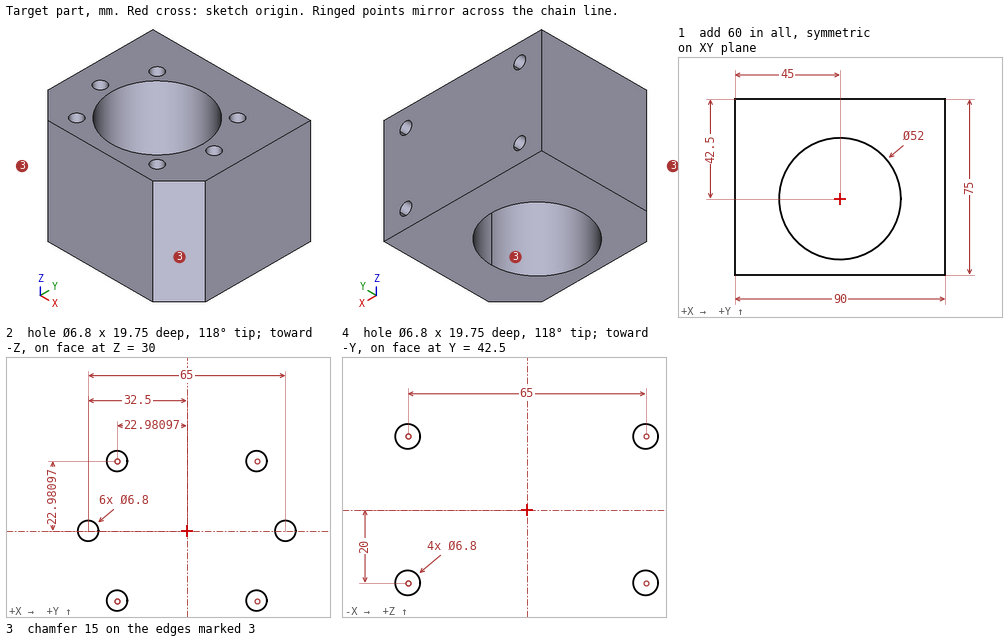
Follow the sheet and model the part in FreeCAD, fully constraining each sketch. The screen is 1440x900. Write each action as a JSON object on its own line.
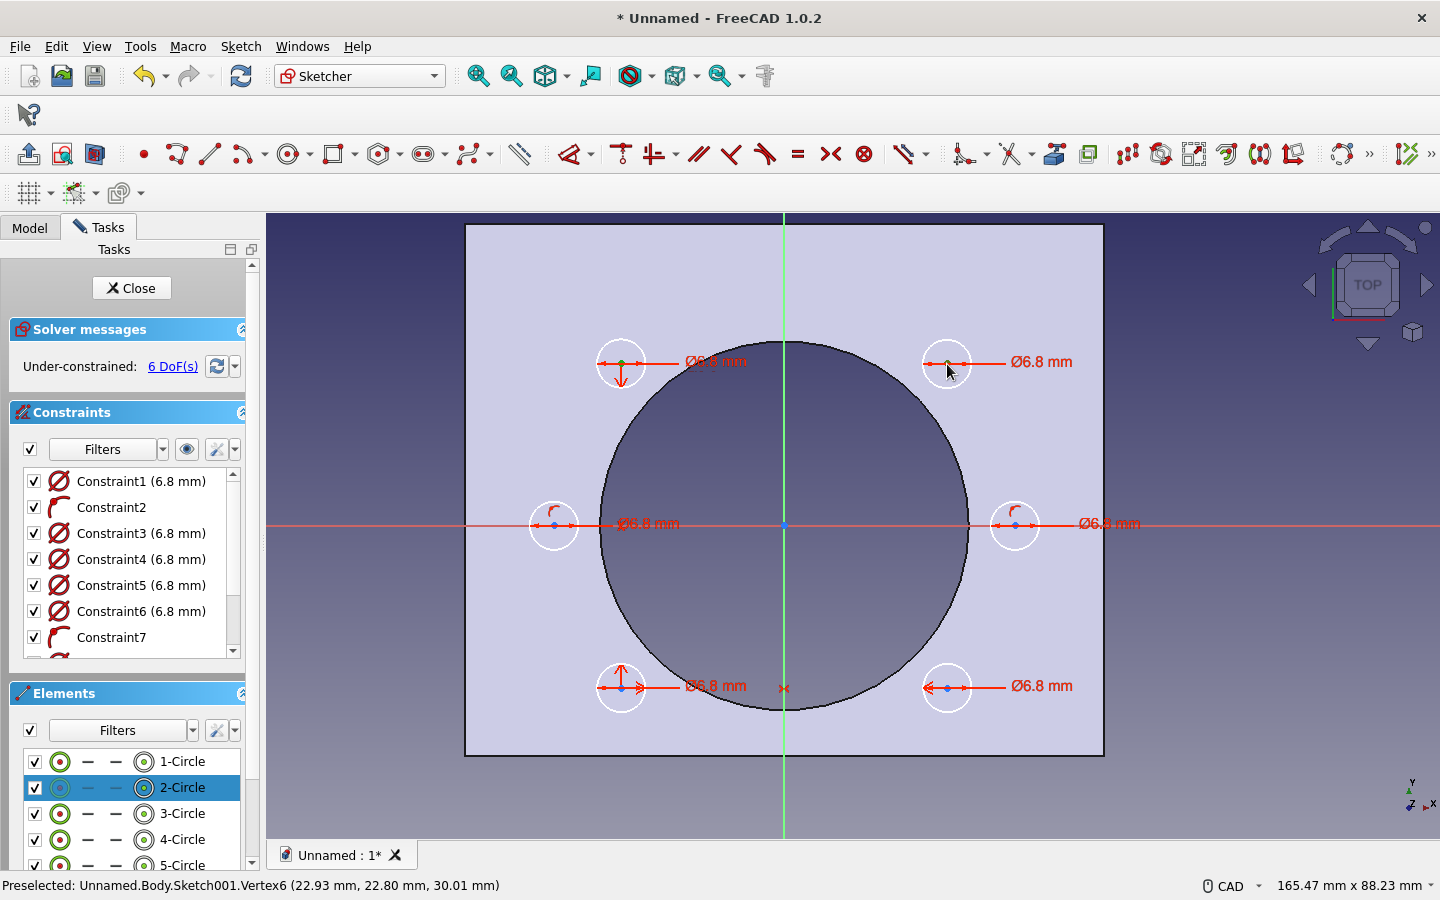
{"action": "left_click", "coordinate": [784, 770]}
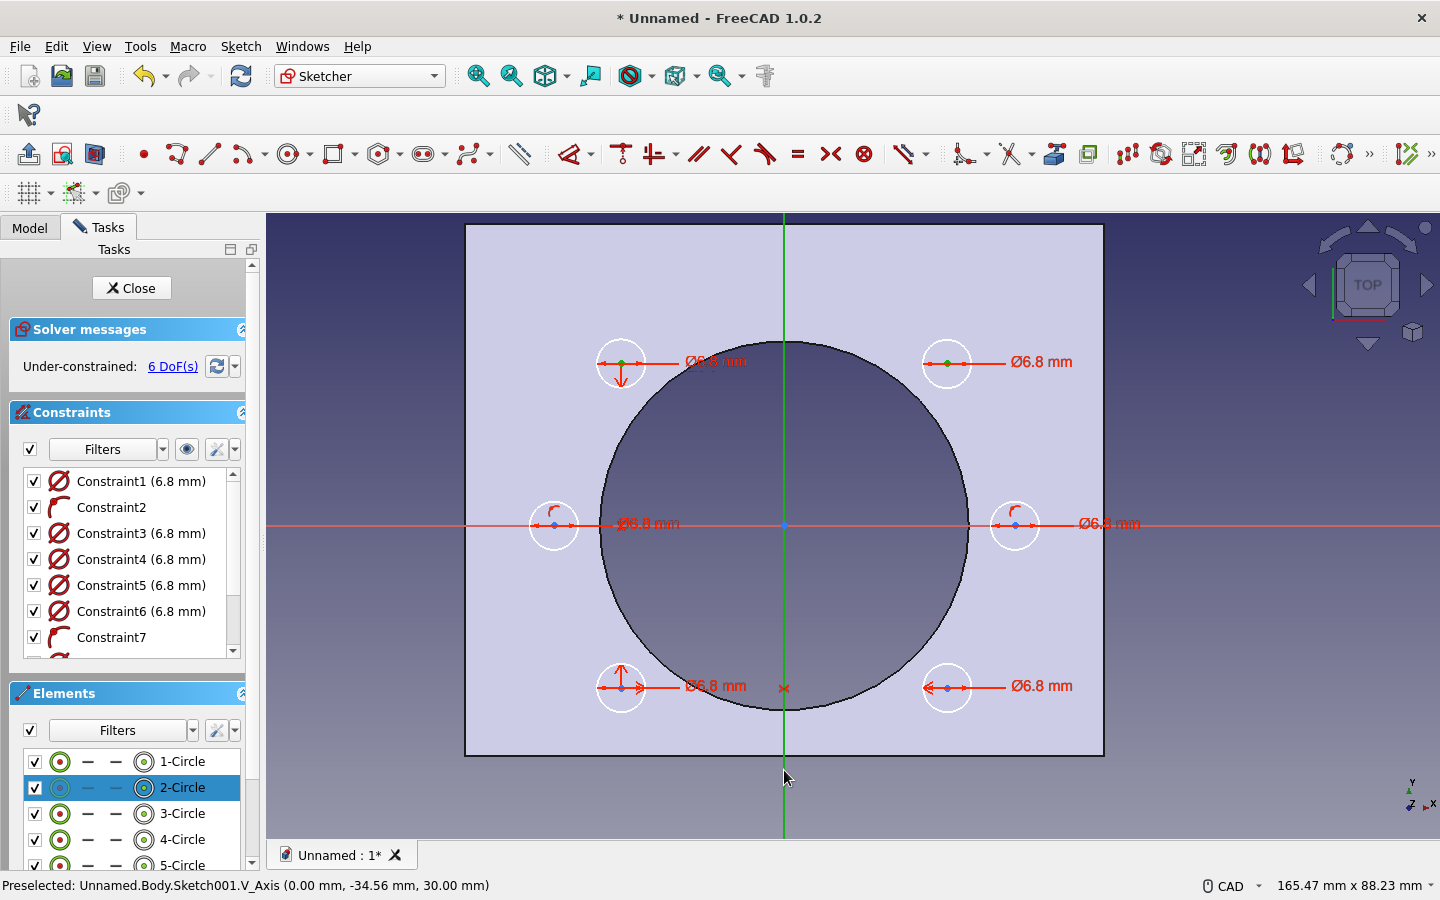
{"action": "left_click", "coordinate": [831, 154]}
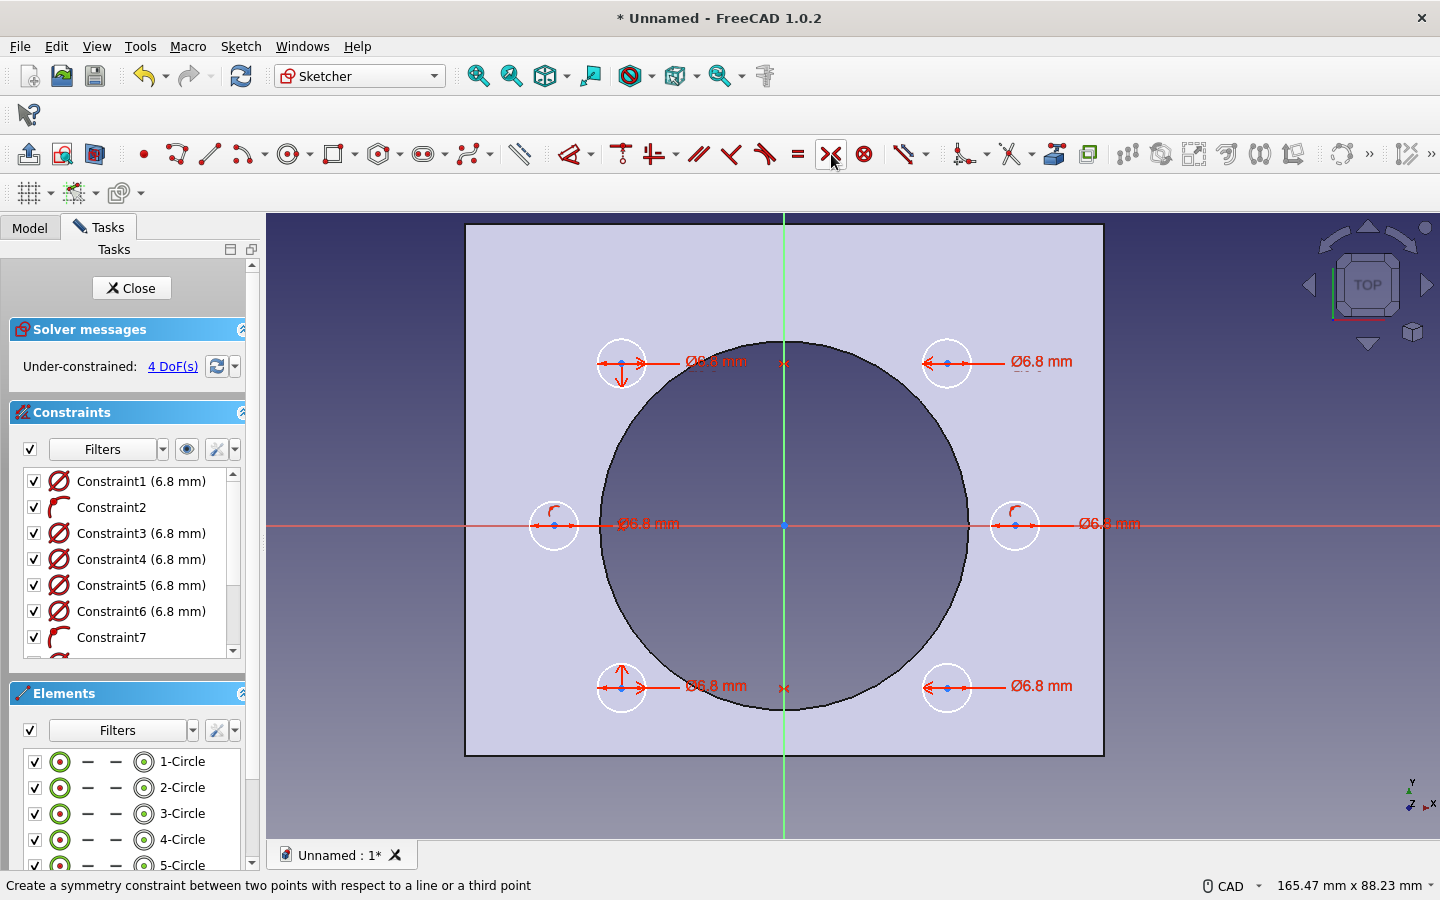
{"action": "left_click", "coordinate": [568, 154]}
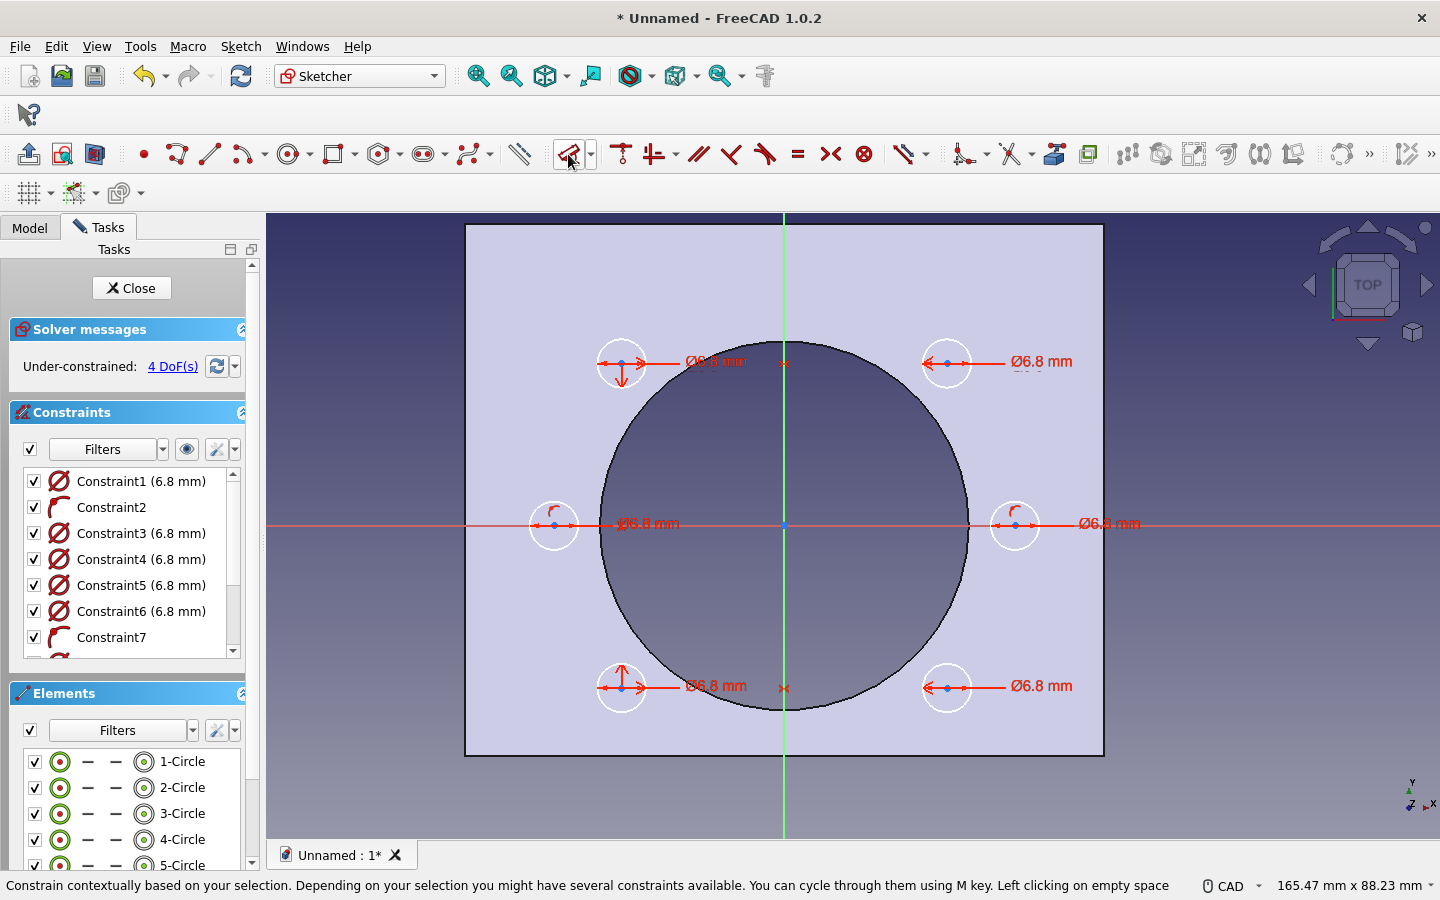
{"action": "left_click", "coordinate": [554, 526]}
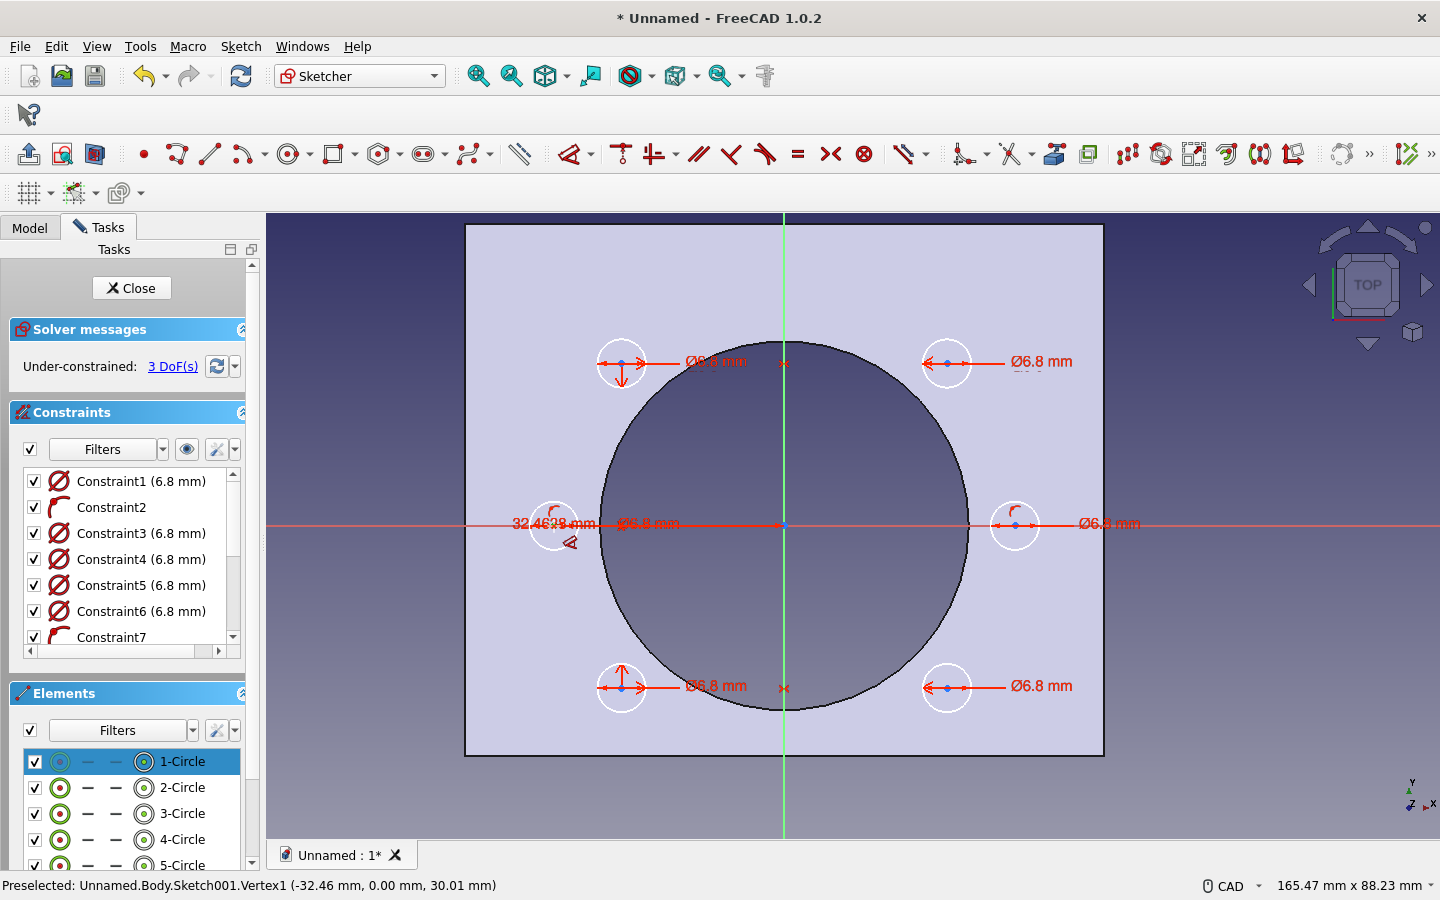
{"action": "left_click", "coordinate": [1015, 526]}
{"action": "left_click", "coordinate": [678, 560]}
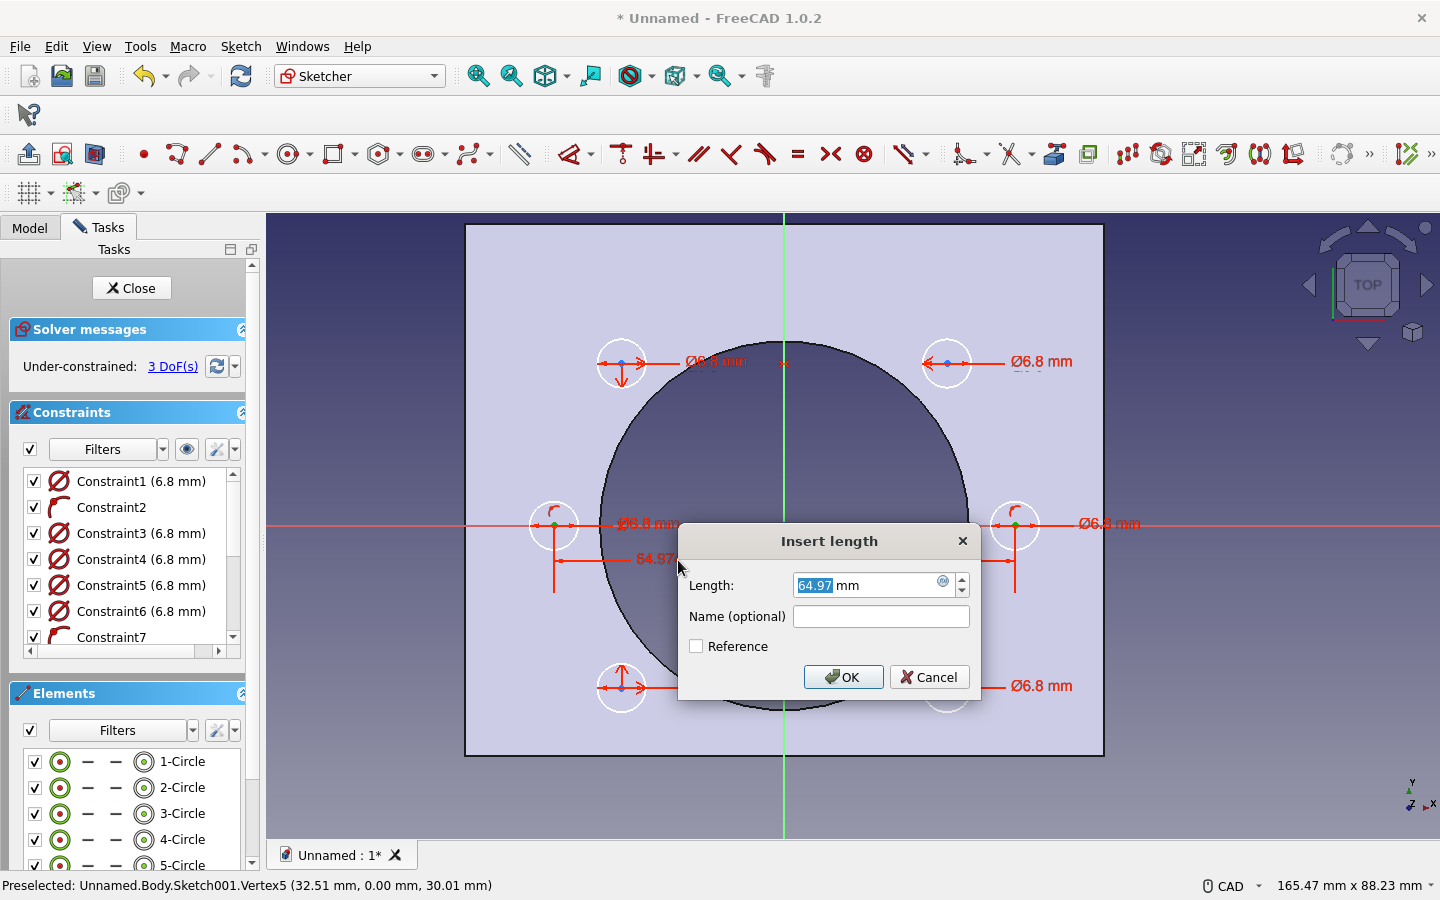
{"action": "type", "text": "65"}
{"action": "key", "text": "Return"}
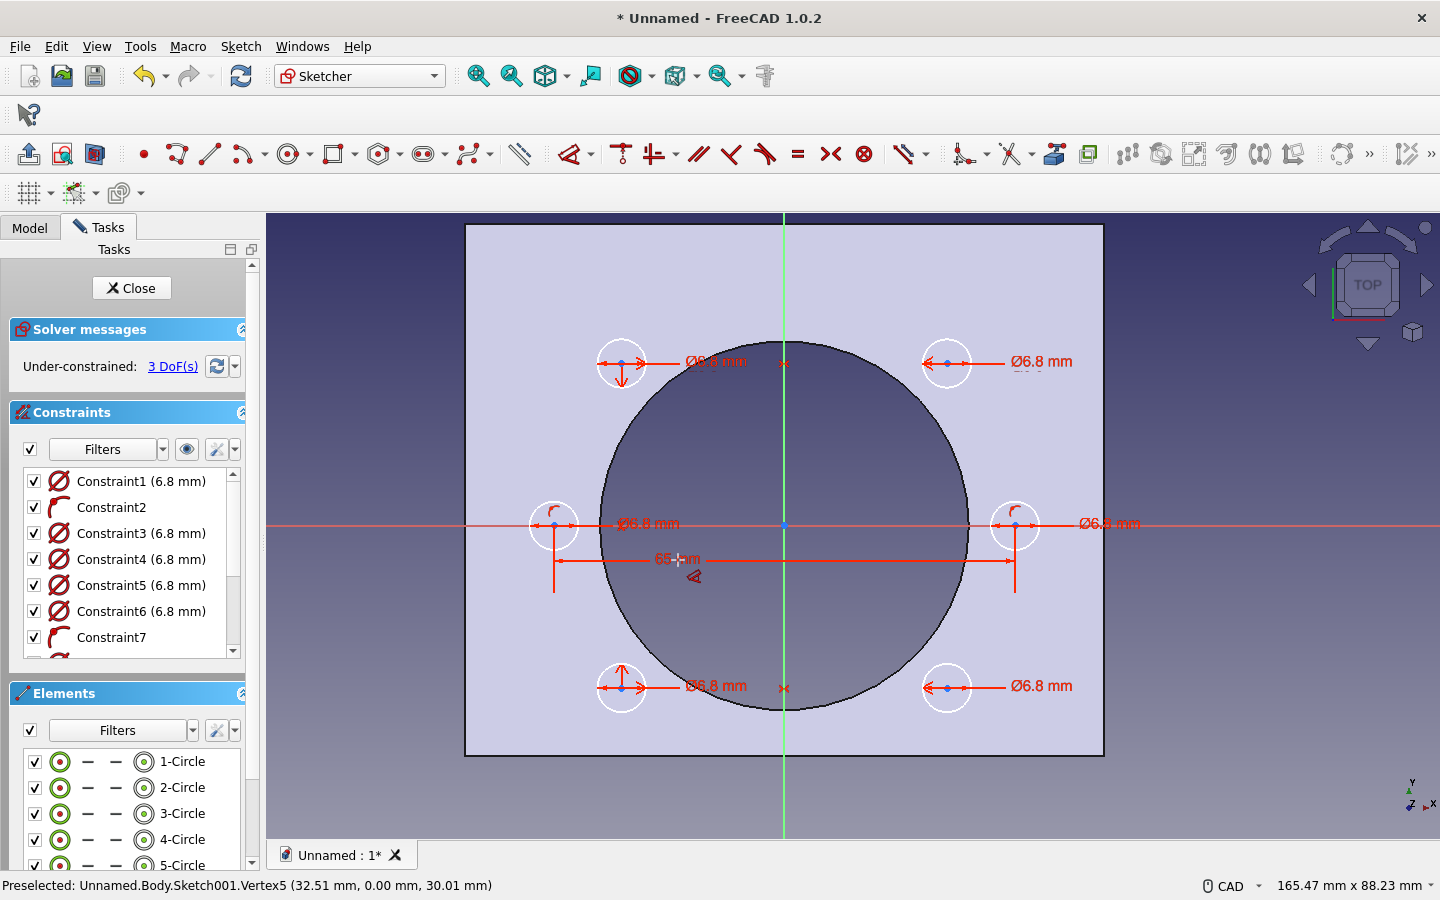
{"action": "left_click", "coordinate": [554, 526]}
{"action": "left_click", "coordinate": [589, 560]}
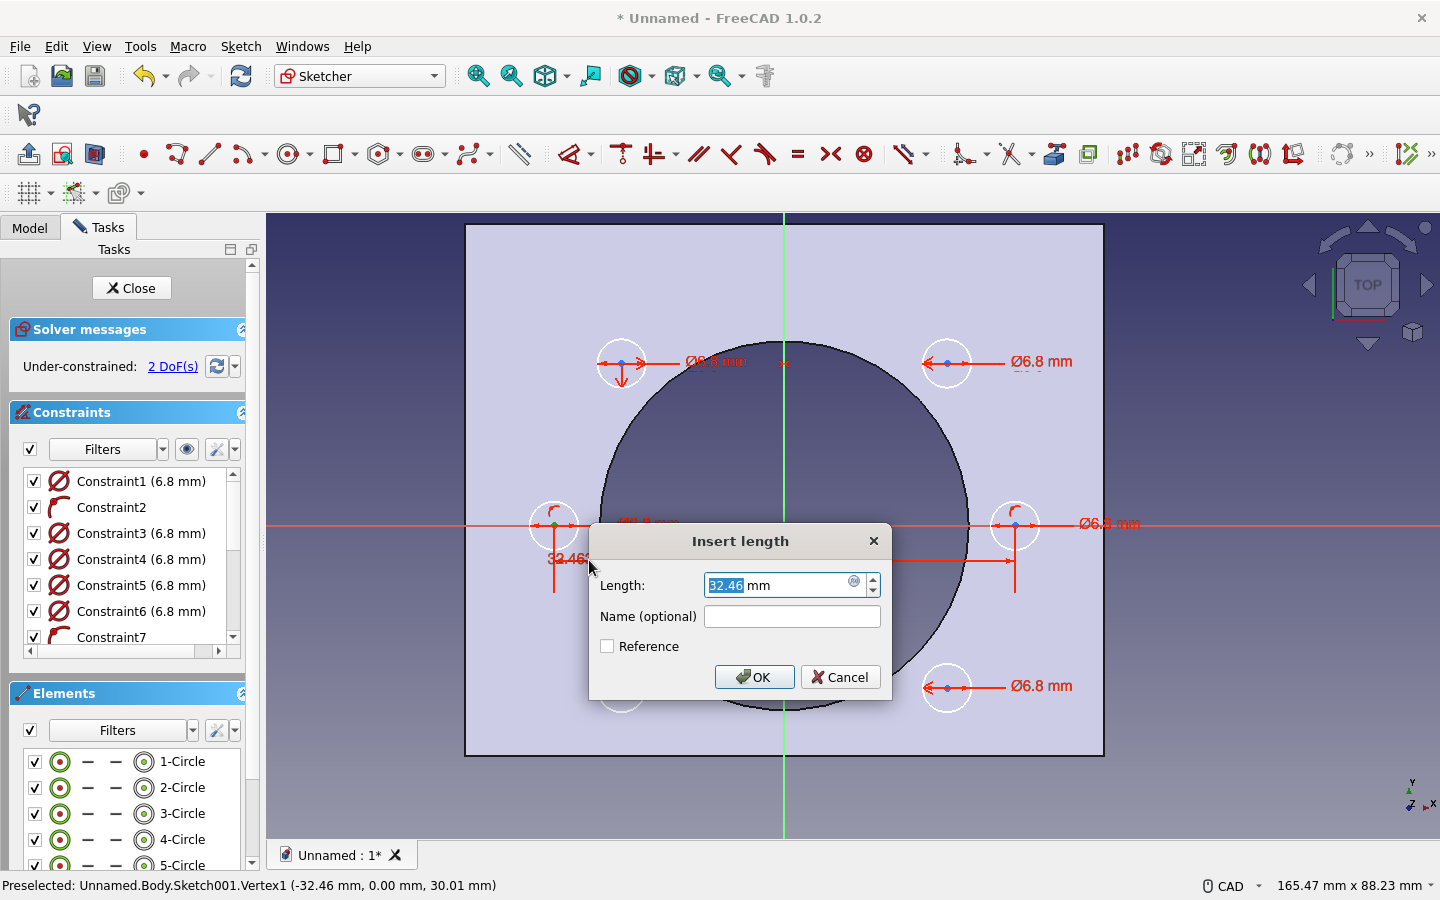
{"action": "type", "text": "32.5"}
{"action": "key", "text": "Return"}